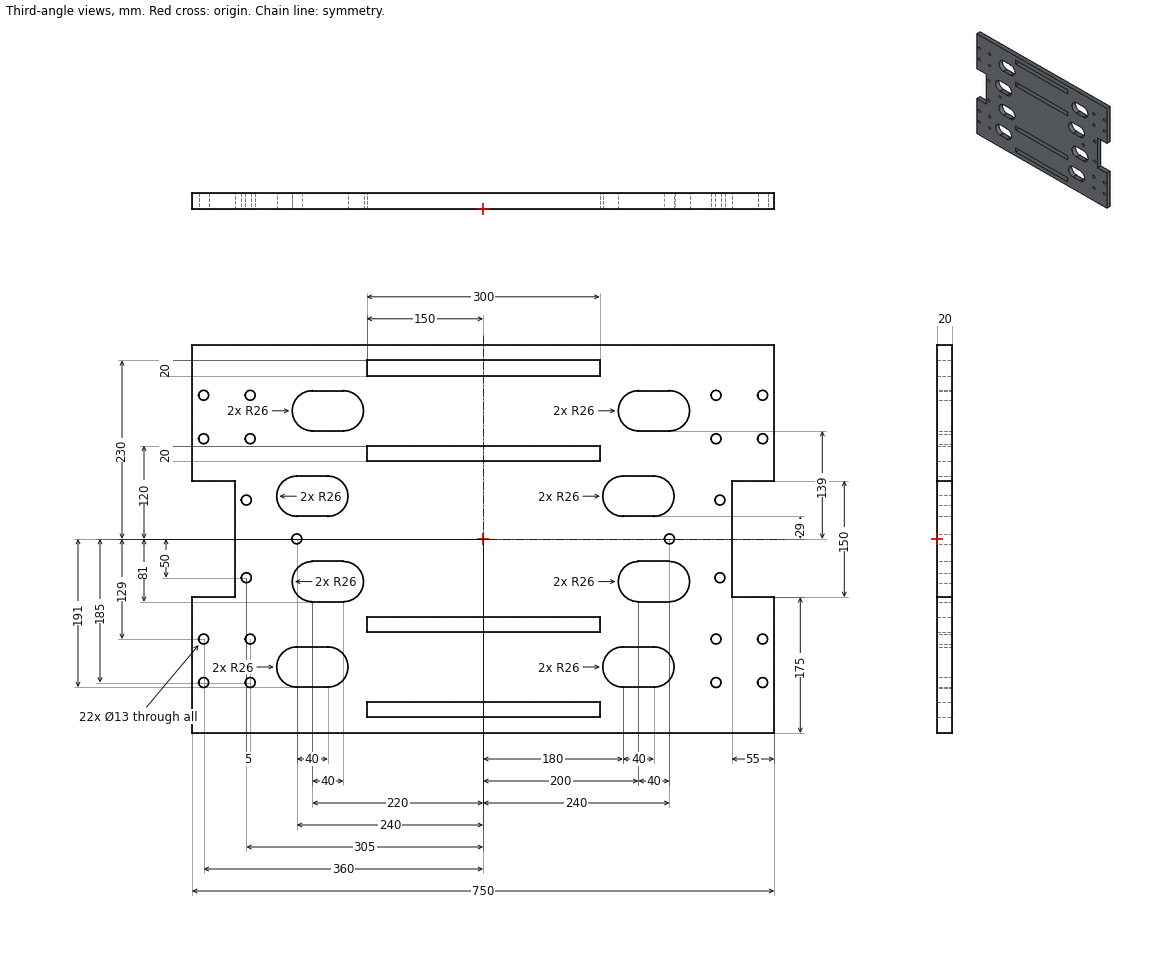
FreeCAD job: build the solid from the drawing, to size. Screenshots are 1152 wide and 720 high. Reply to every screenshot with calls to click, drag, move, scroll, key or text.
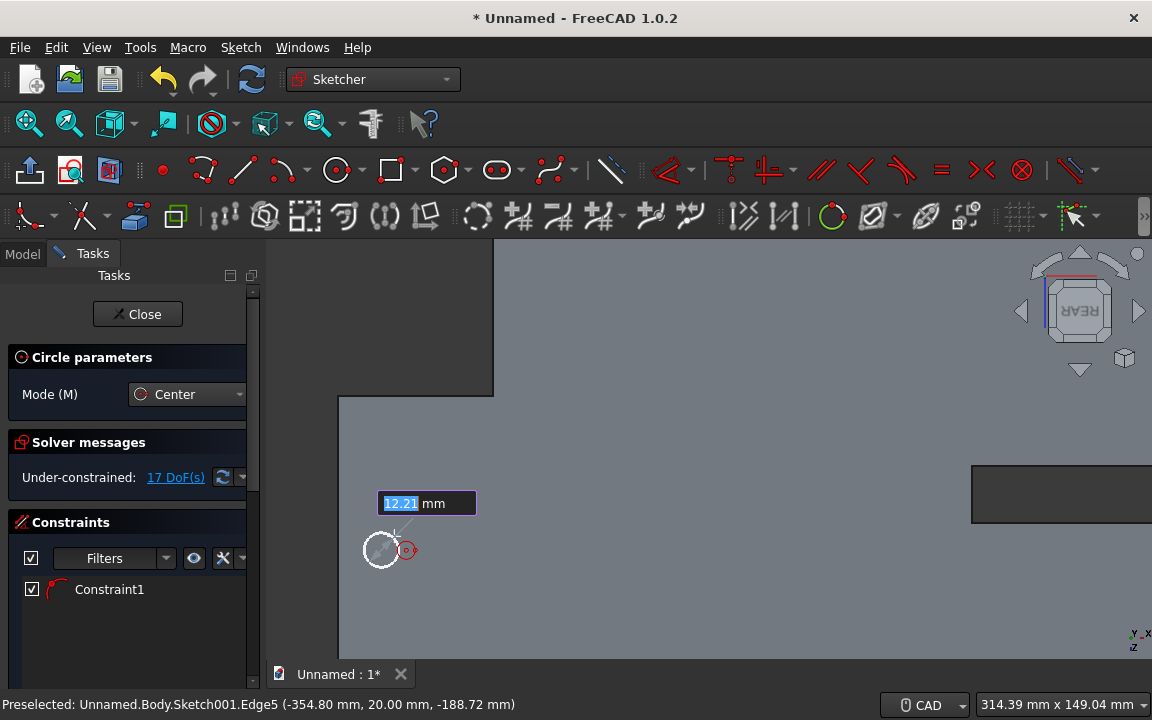
click(393, 535)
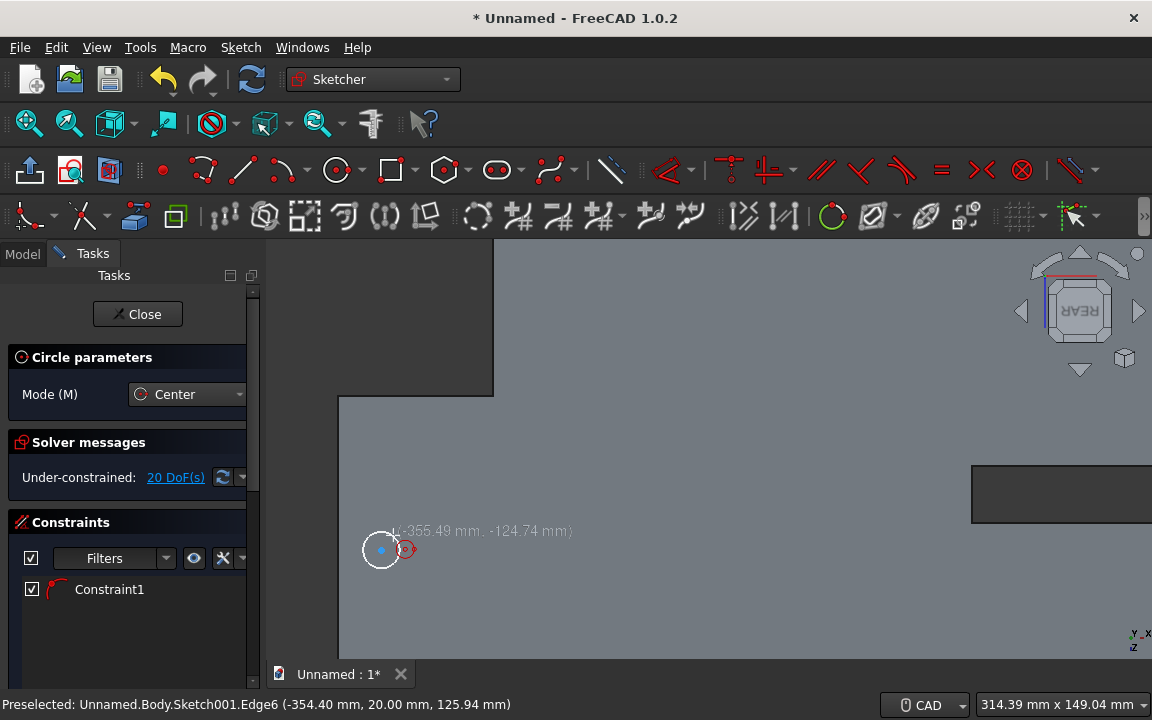
scroll(394, 536, down, 7)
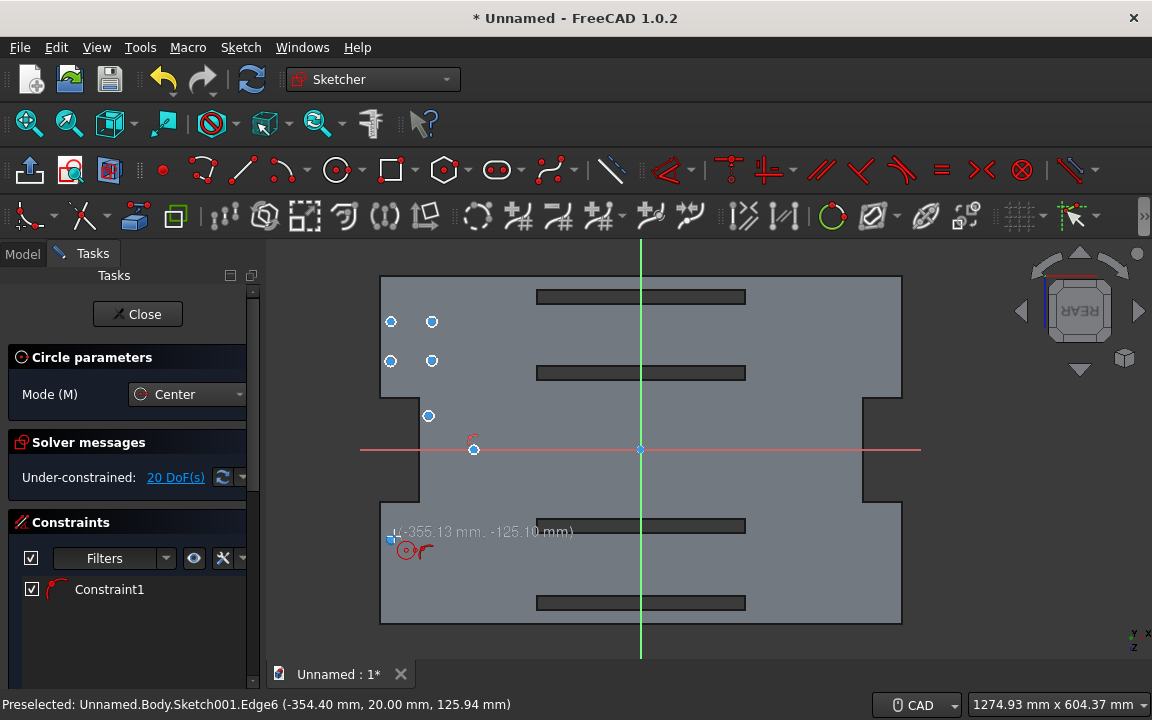
scroll(391, 578, up, 9)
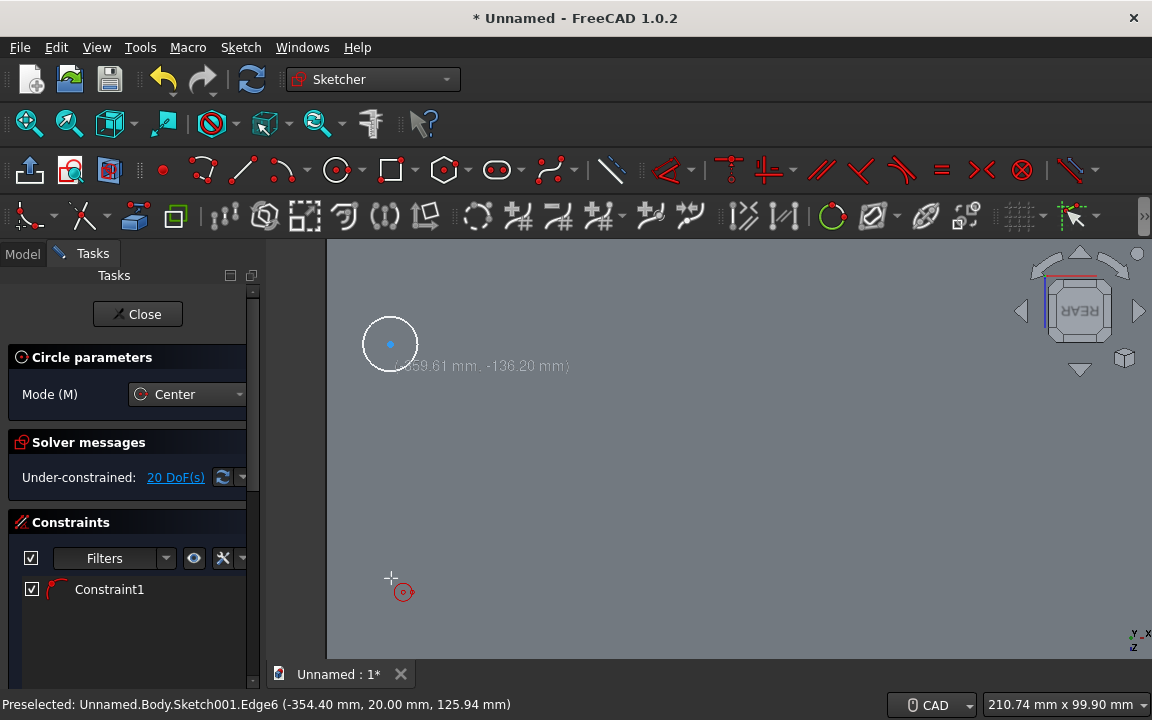
scroll(391, 578, down, 9)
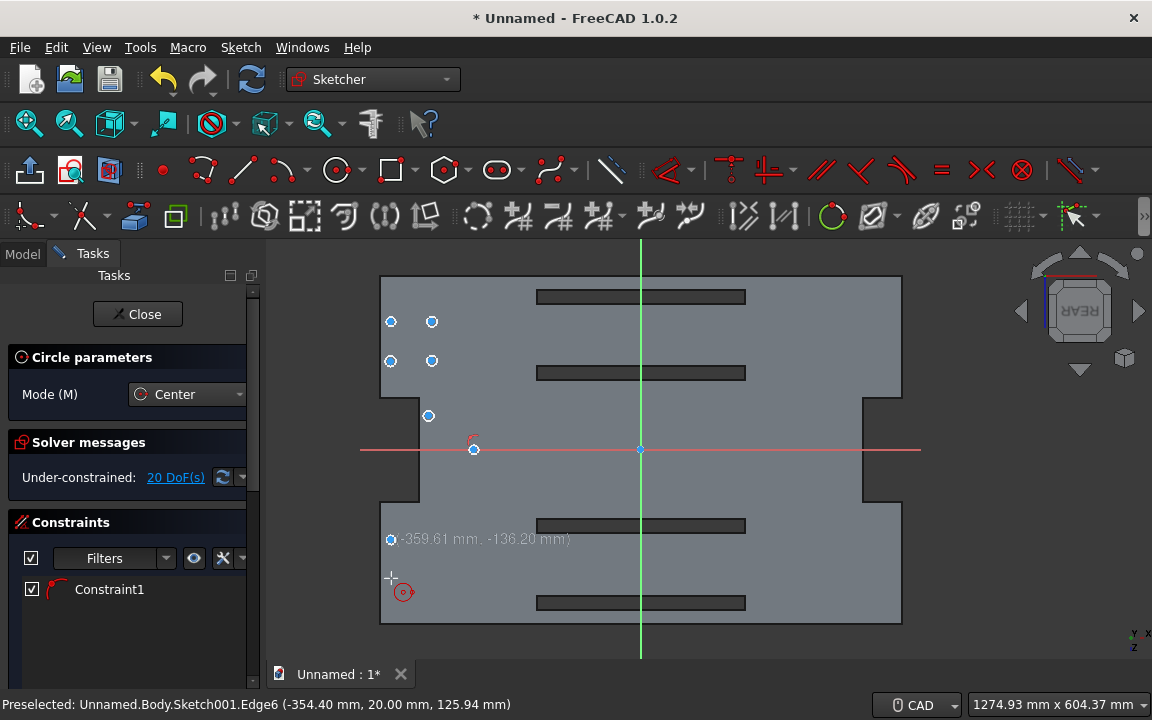
click(391, 578)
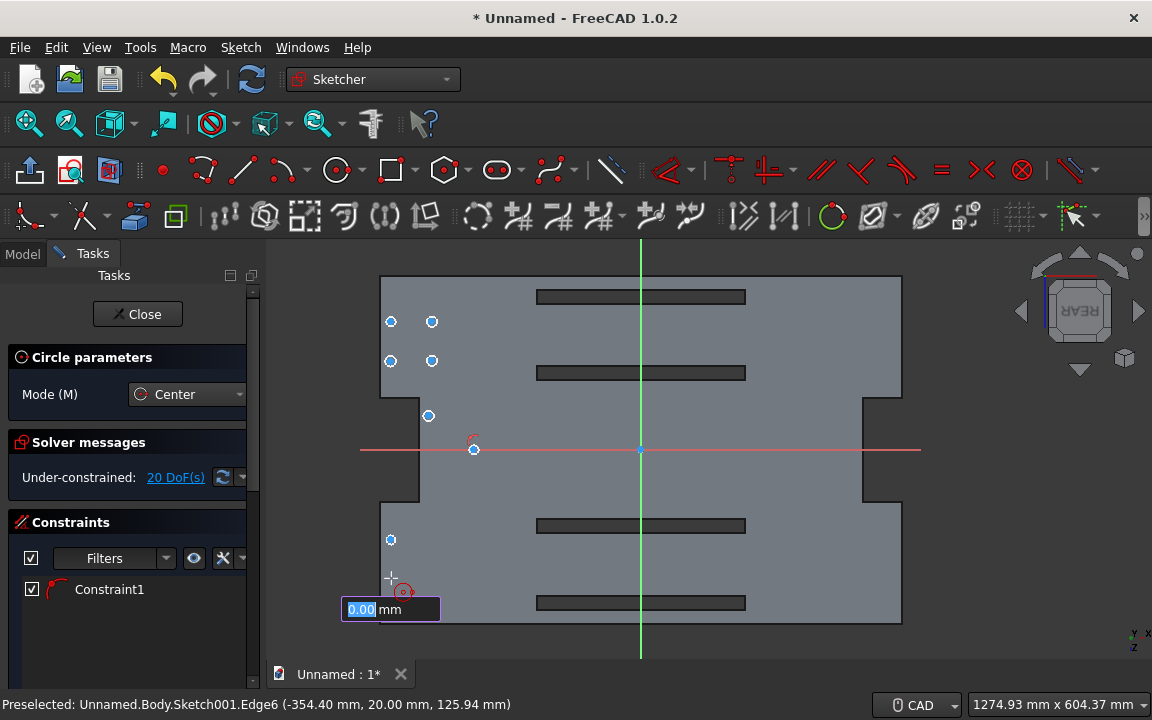
scroll(394, 575, up, 7)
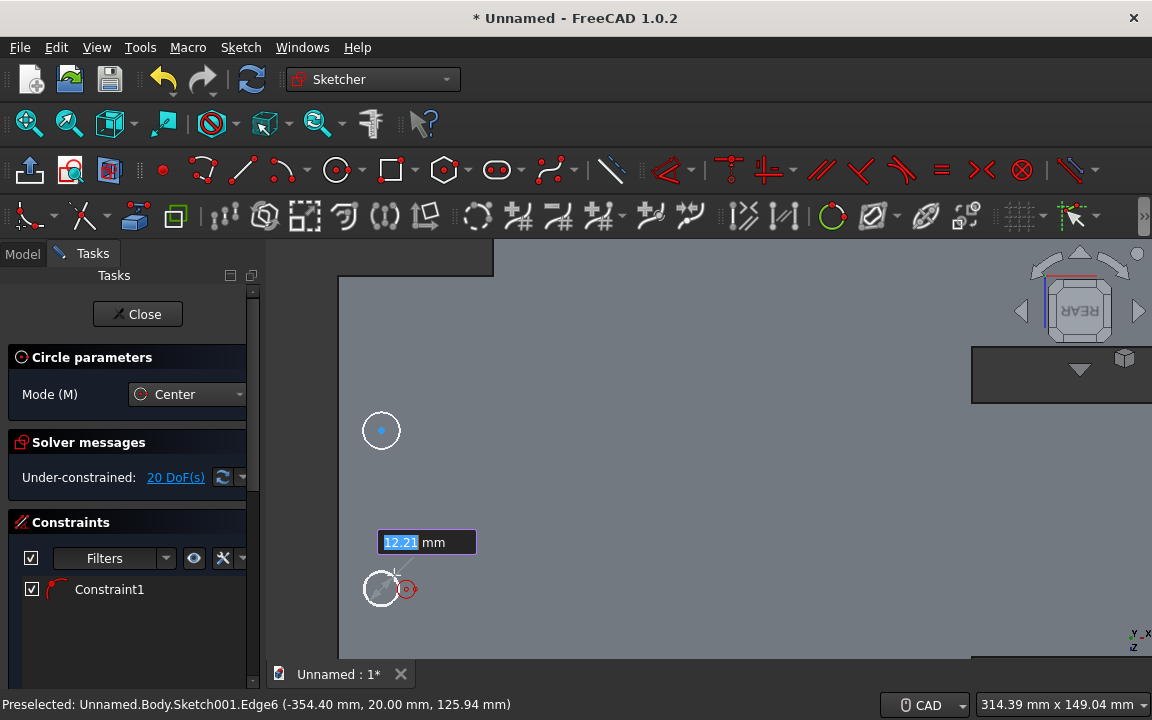
click(393, 573)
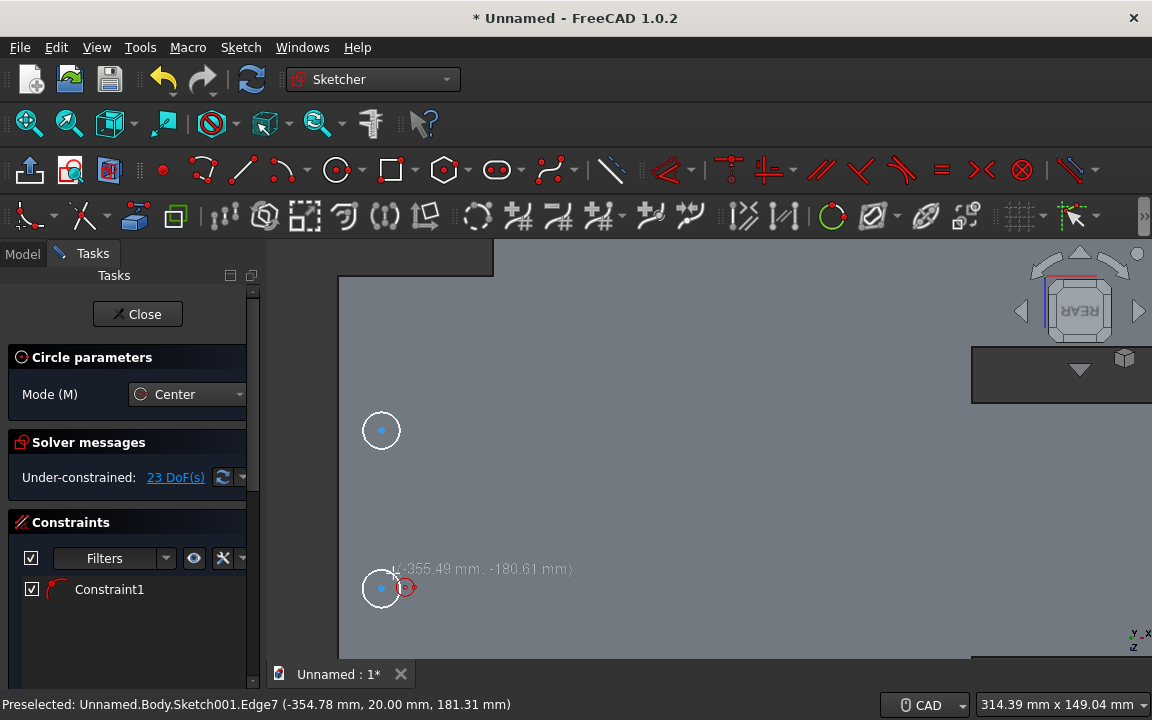
scroll(549, 429, up, 2)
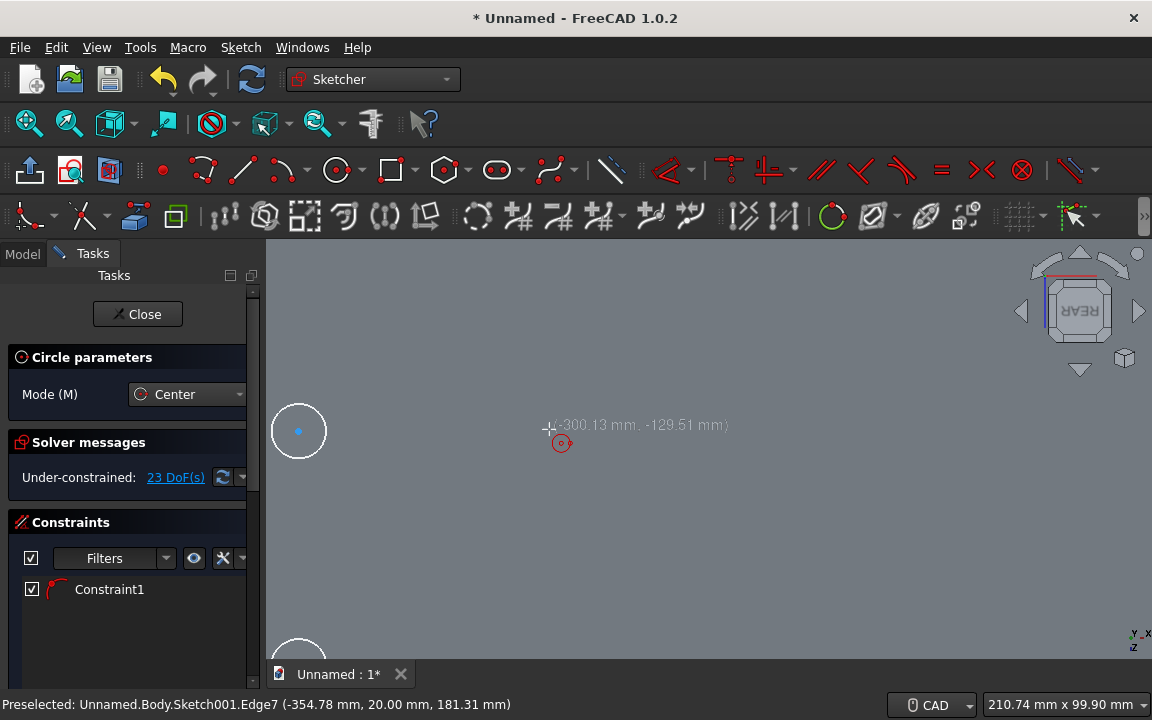
scroll(409, 561, down, 9)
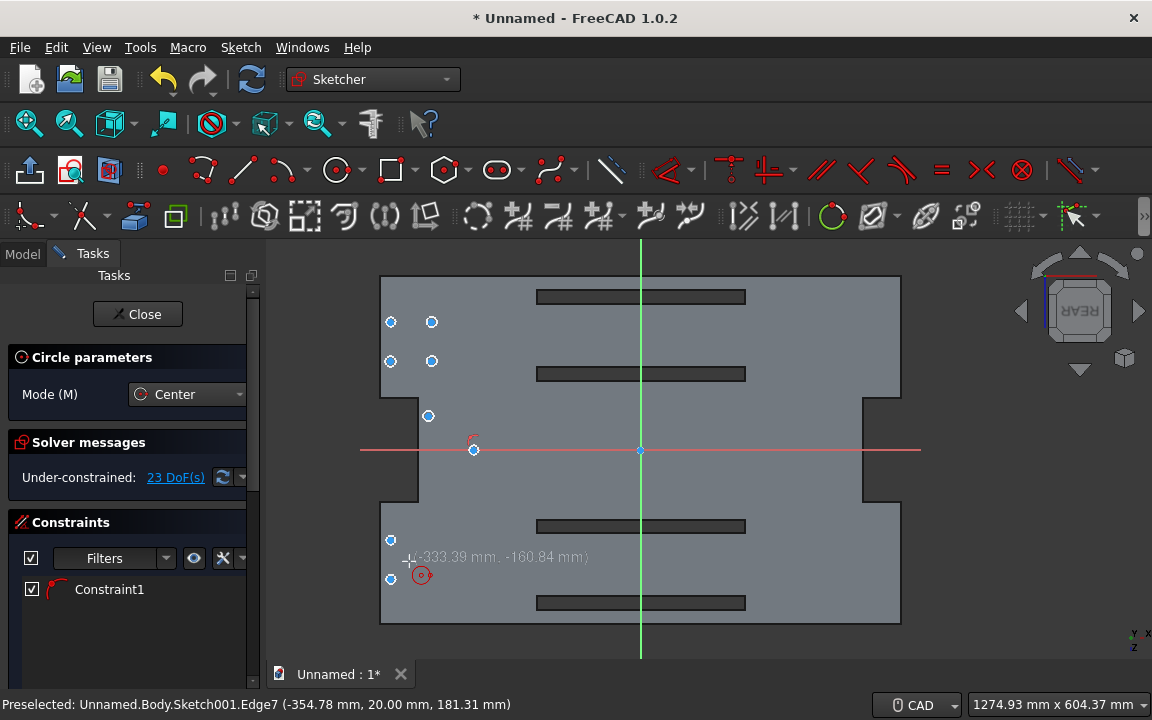
click(432, 540)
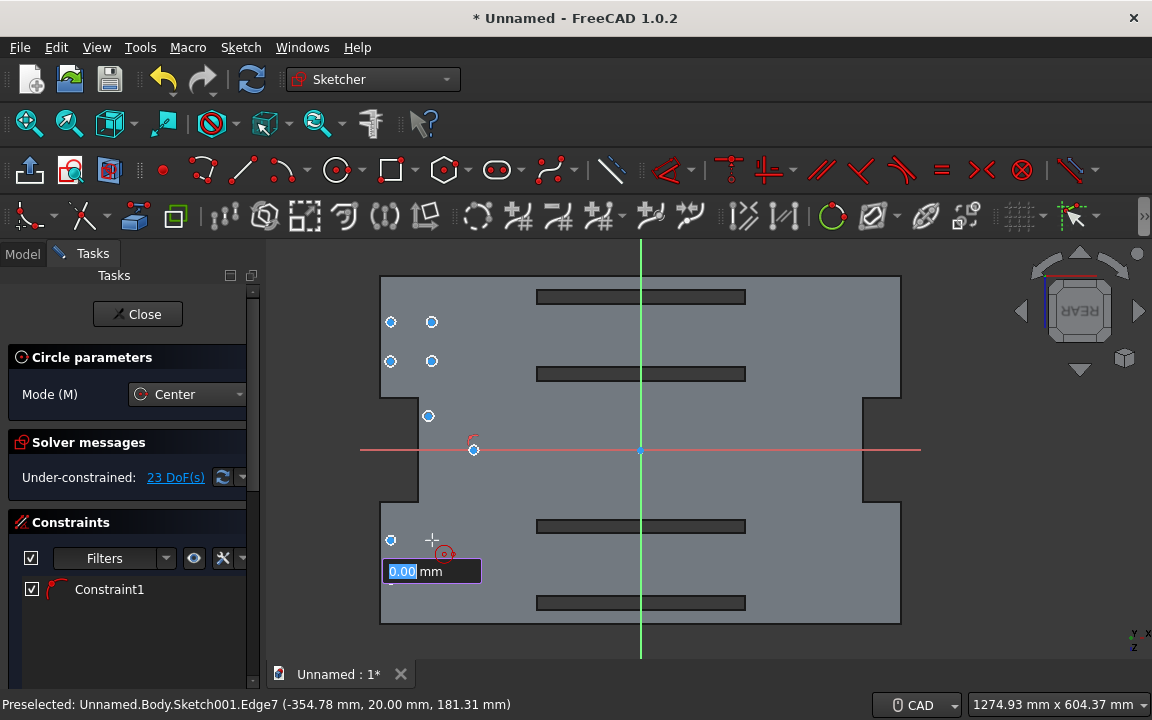
scroll(436, 536, up, 7)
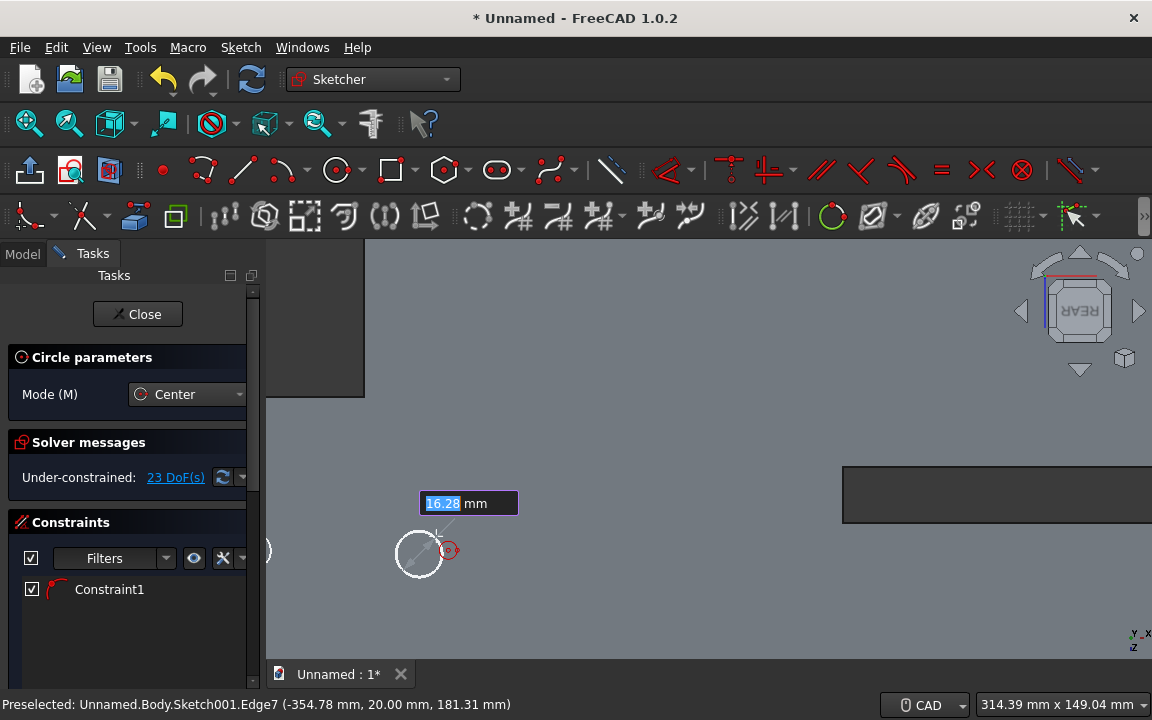
click(434, 536)